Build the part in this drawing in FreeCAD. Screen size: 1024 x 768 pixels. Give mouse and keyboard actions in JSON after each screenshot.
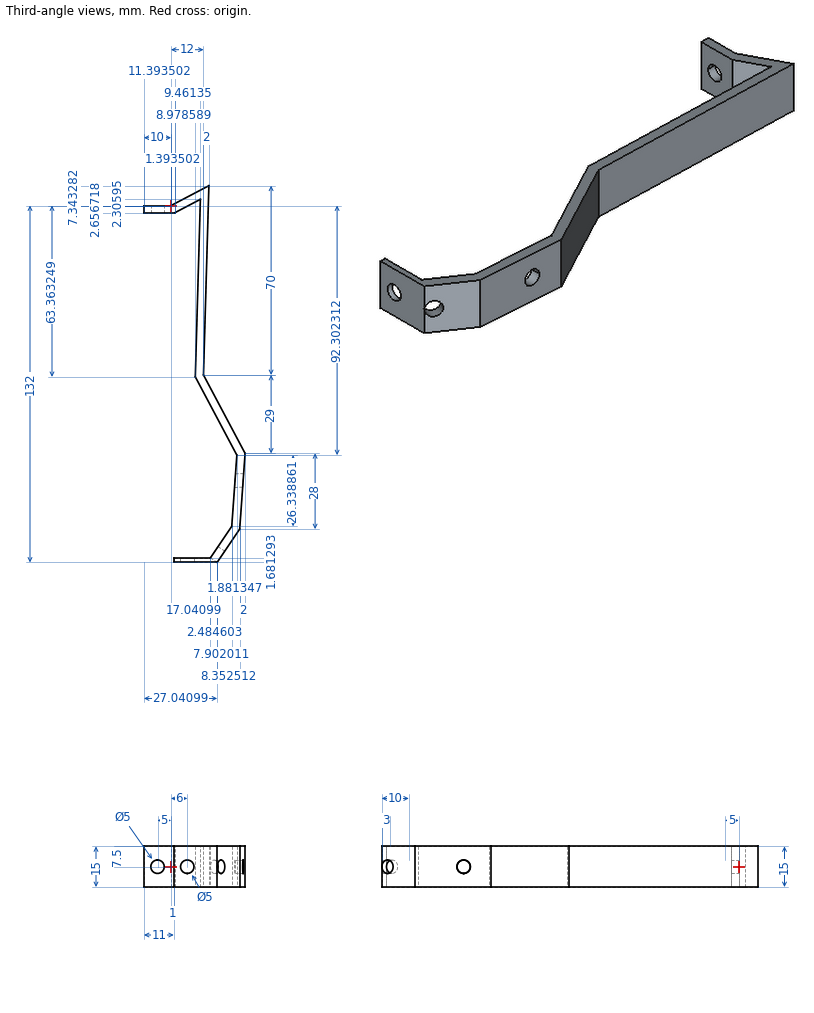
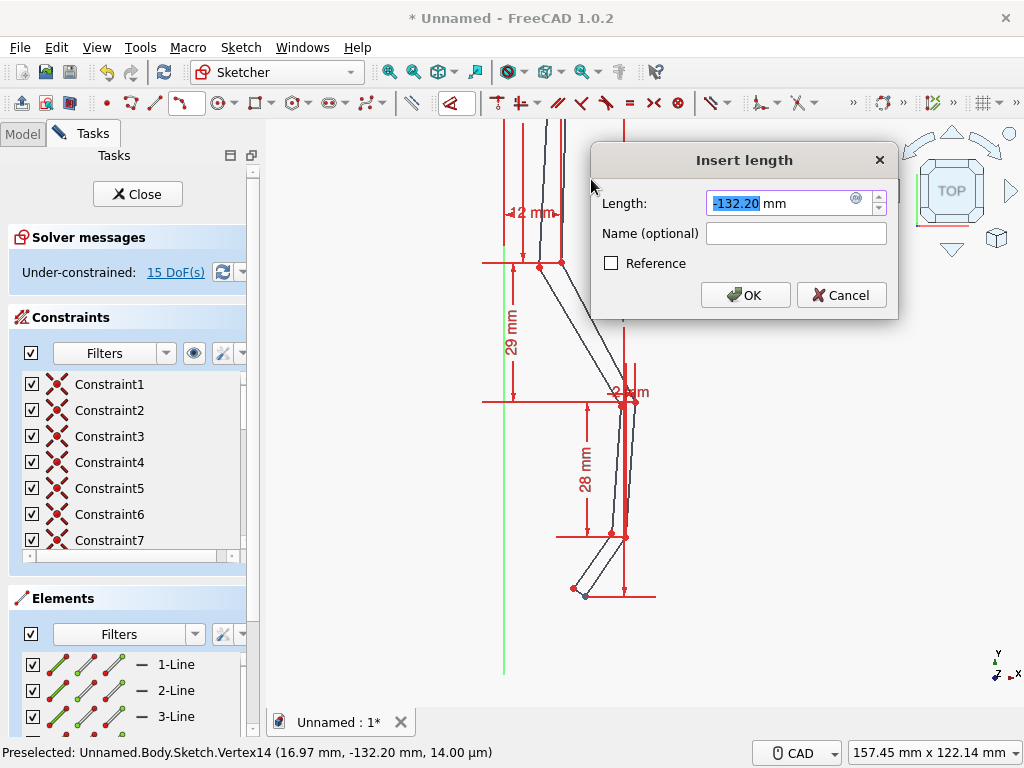
{"action": "type", "text": "-132"}
{"action": "key", "text": "Return"}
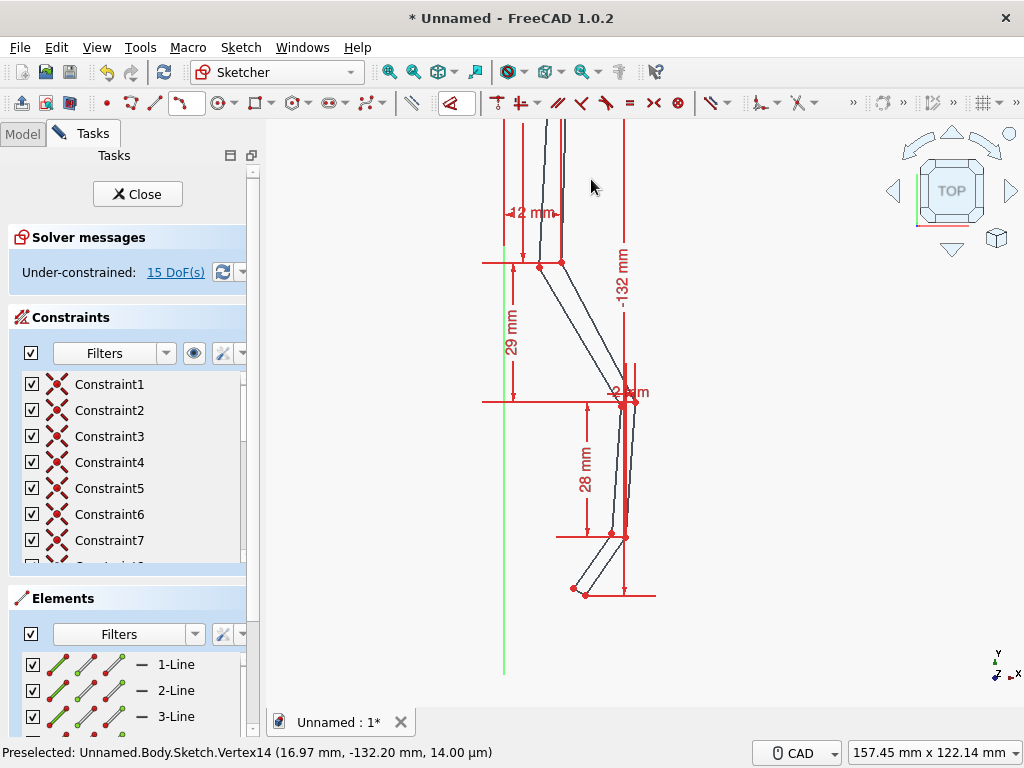
{"action": "scroll", "coordinate": [585, 599], "scroll_direction": "down", "scroll_amount": 3}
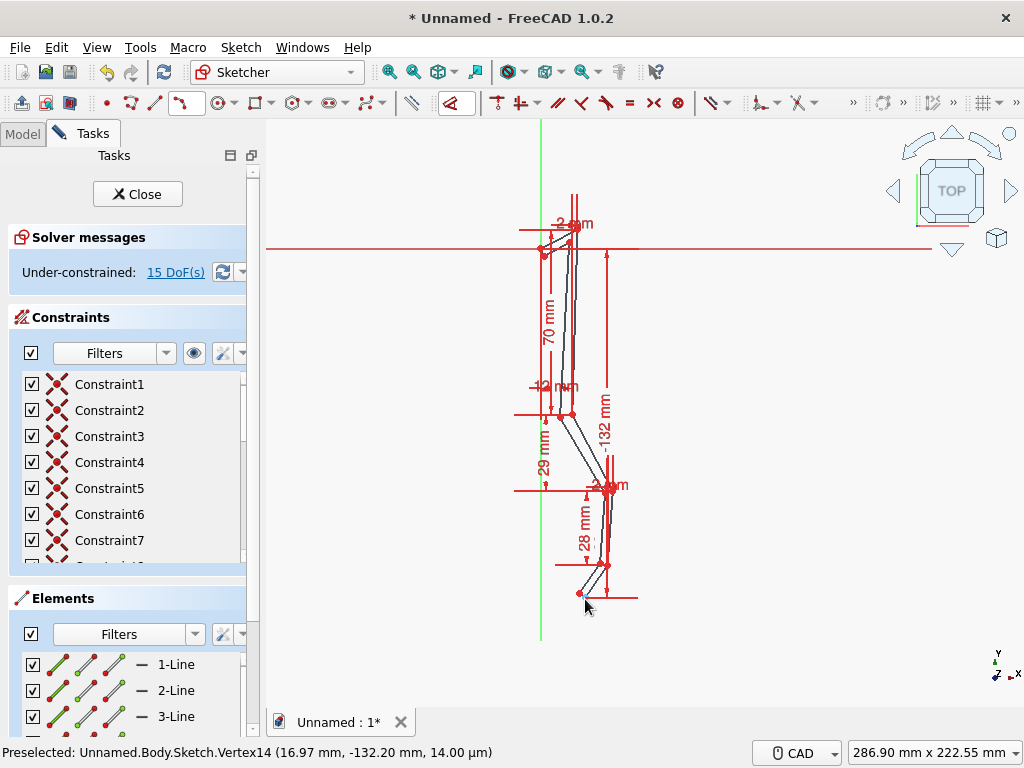
{"action": "scroll", "coordinate": [569, 243], "scroll_direction": "up", "scroll_amount": 10}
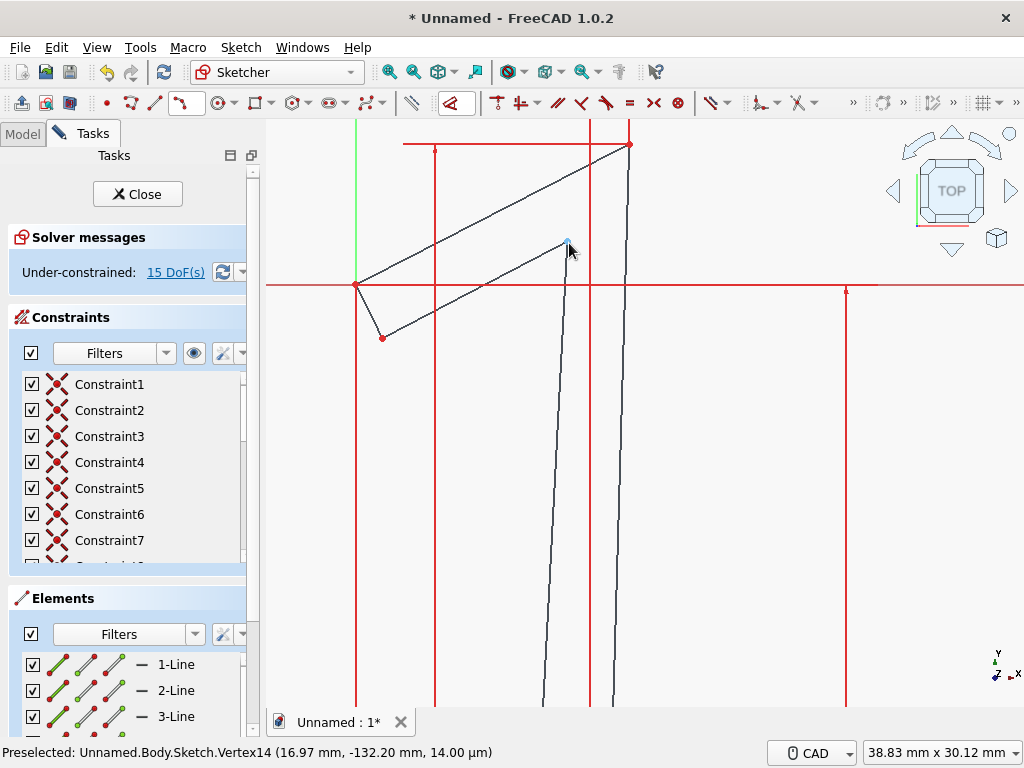
{"action": "left_click", "coordinate": [567, 241]}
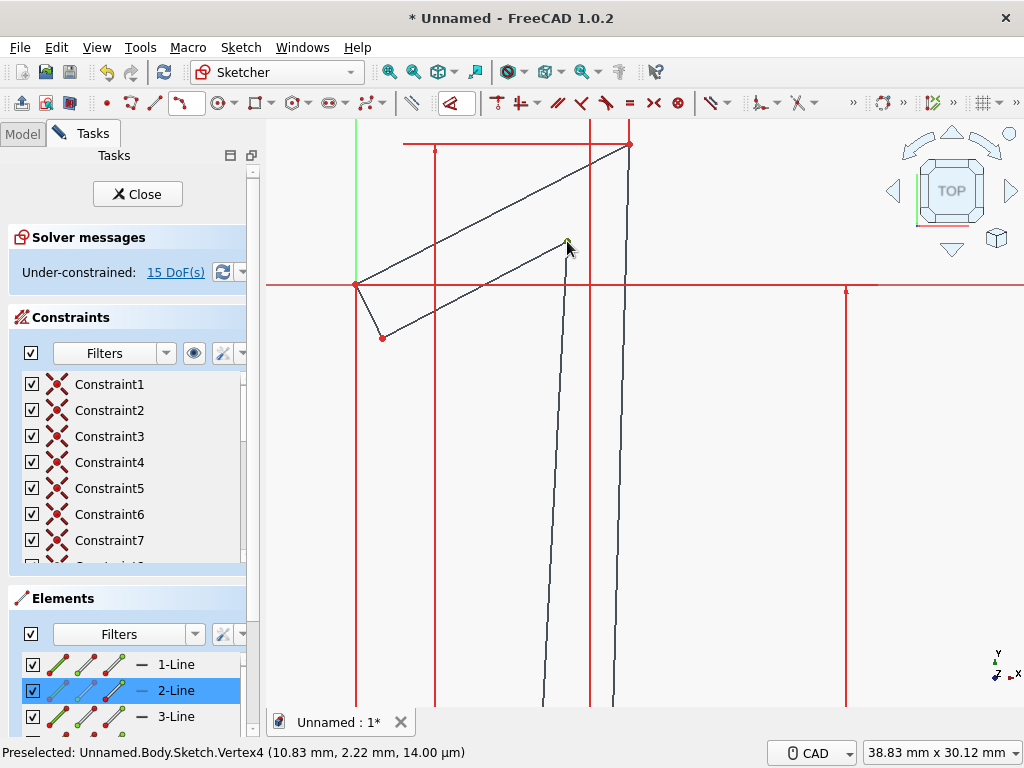
{"action": "key", "text": "i"}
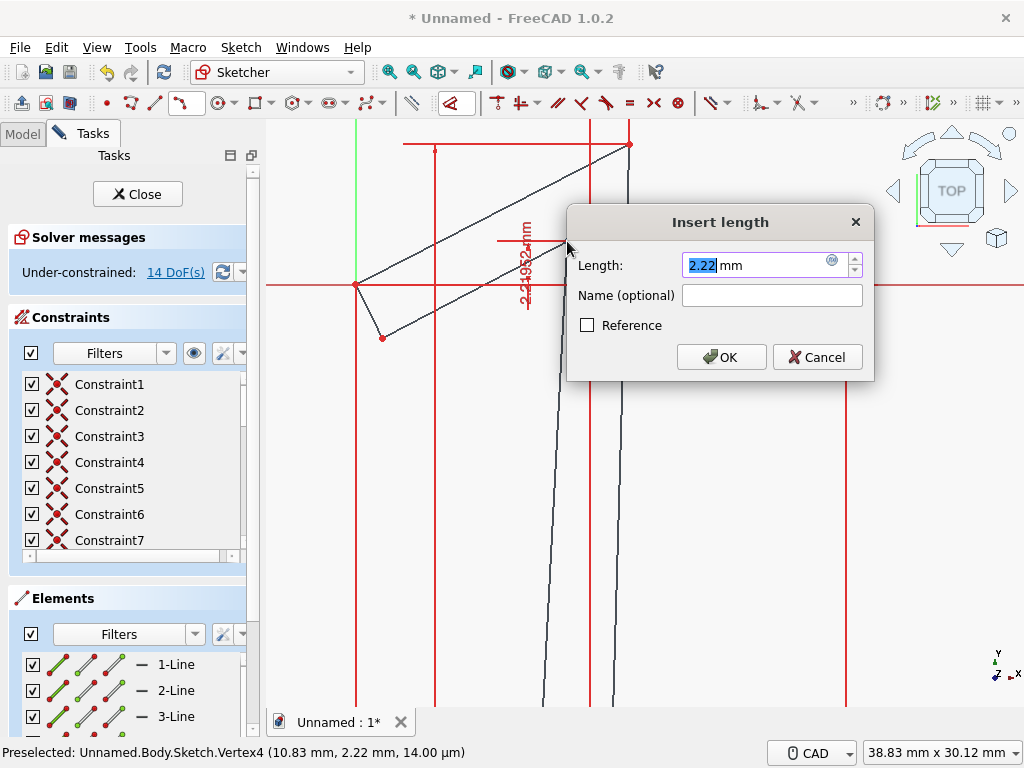
{"action": "type", "text": "2.30595"}
{"action": "key", "text": "Return"}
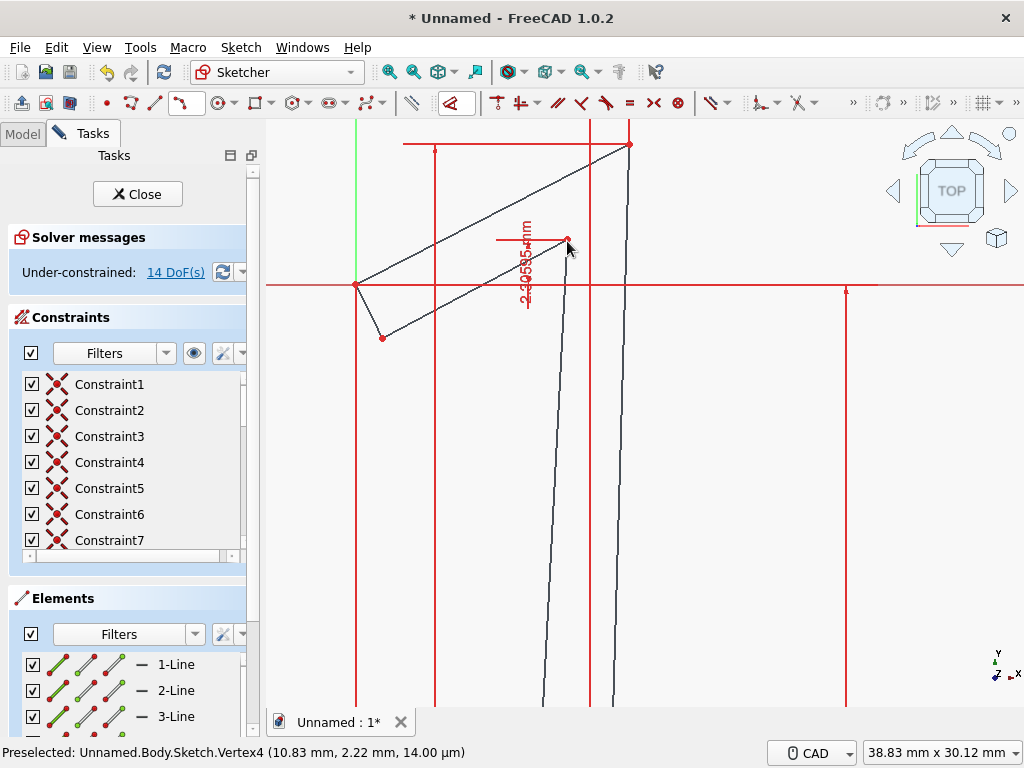
{"action": "left_click", "coordinate": [438, 309]}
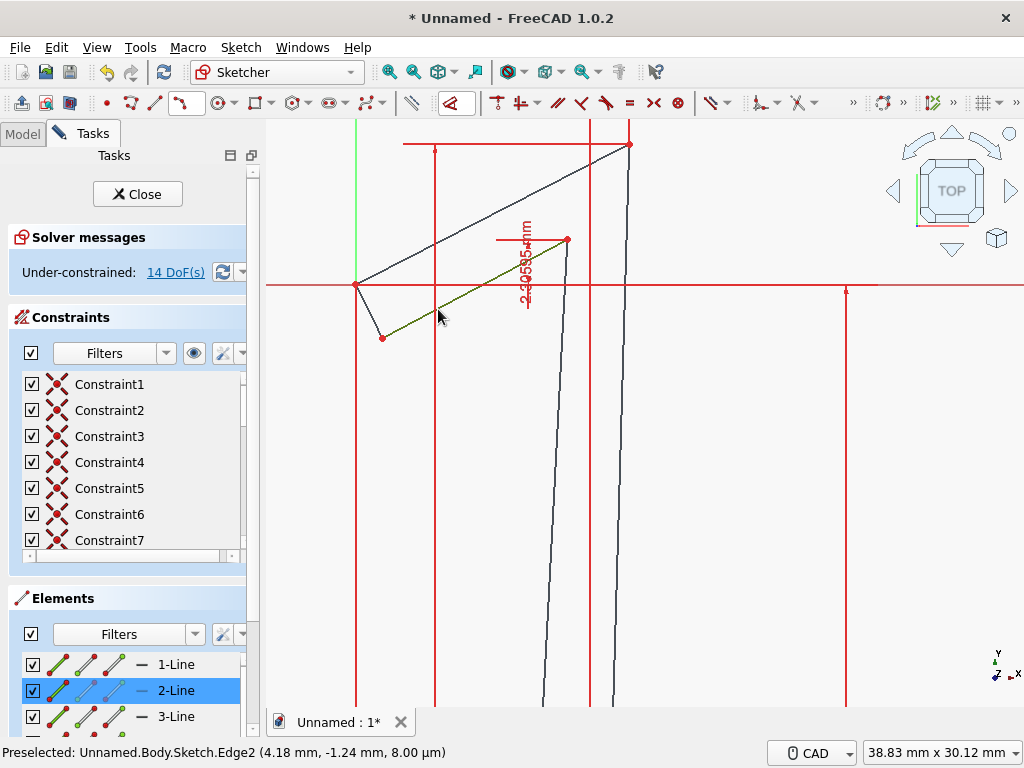
{"action": "key", "text": "l"}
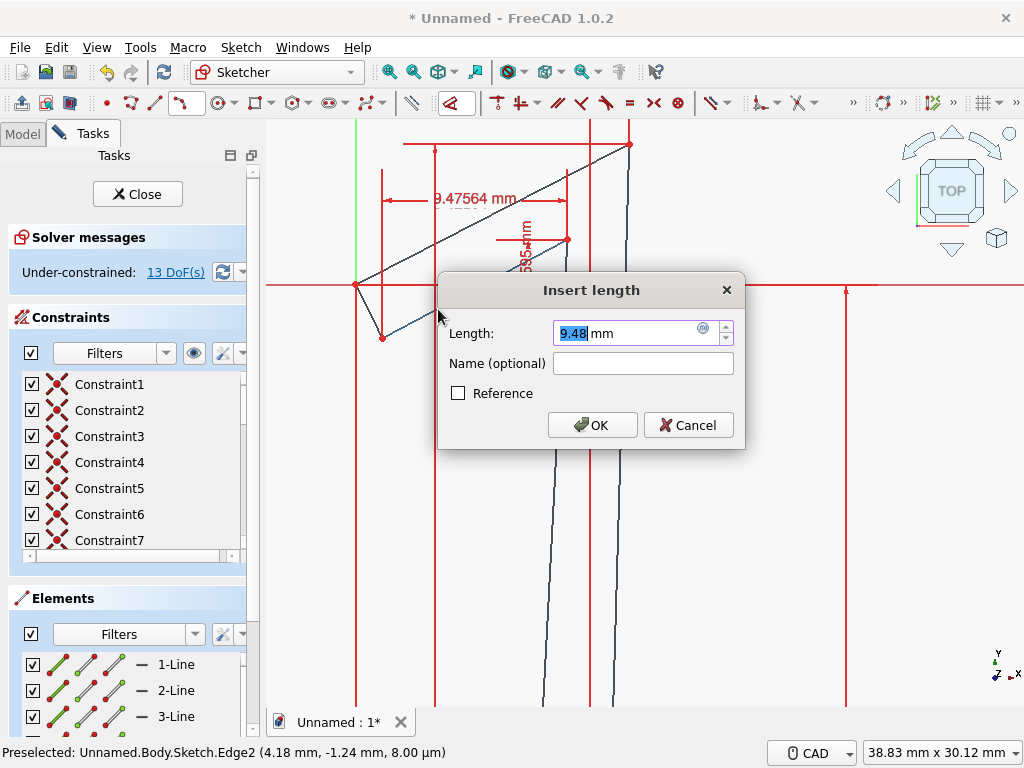
{"action": "type", "text": "9.46135"}
{"action": "key", "text": "Return"}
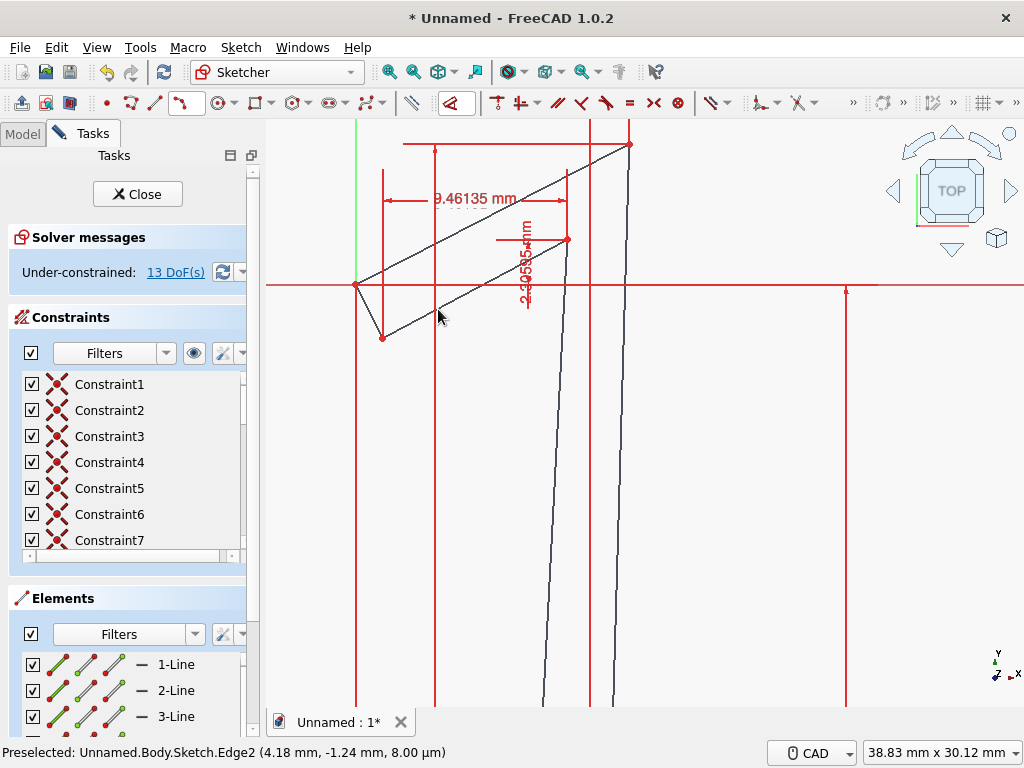
{"action": "scroll", "coordinate": [383, 338], "scroll_direction": "up", "scroll_amount": 2}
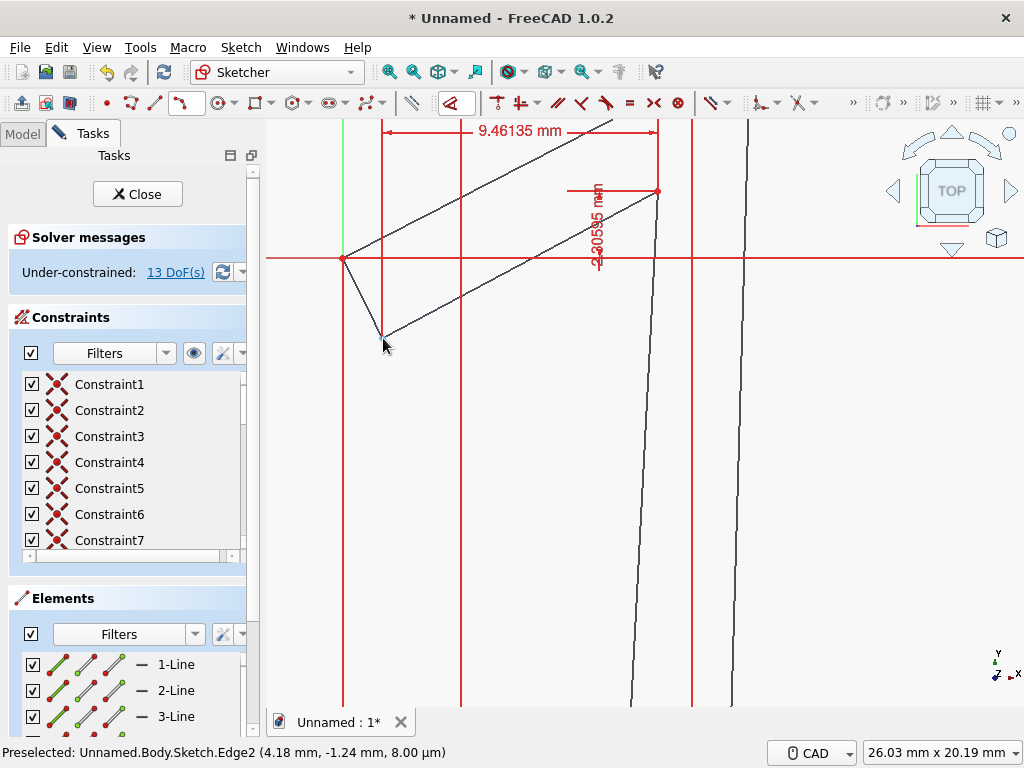
{"action": "left_click", "coordinate": [382, 338]}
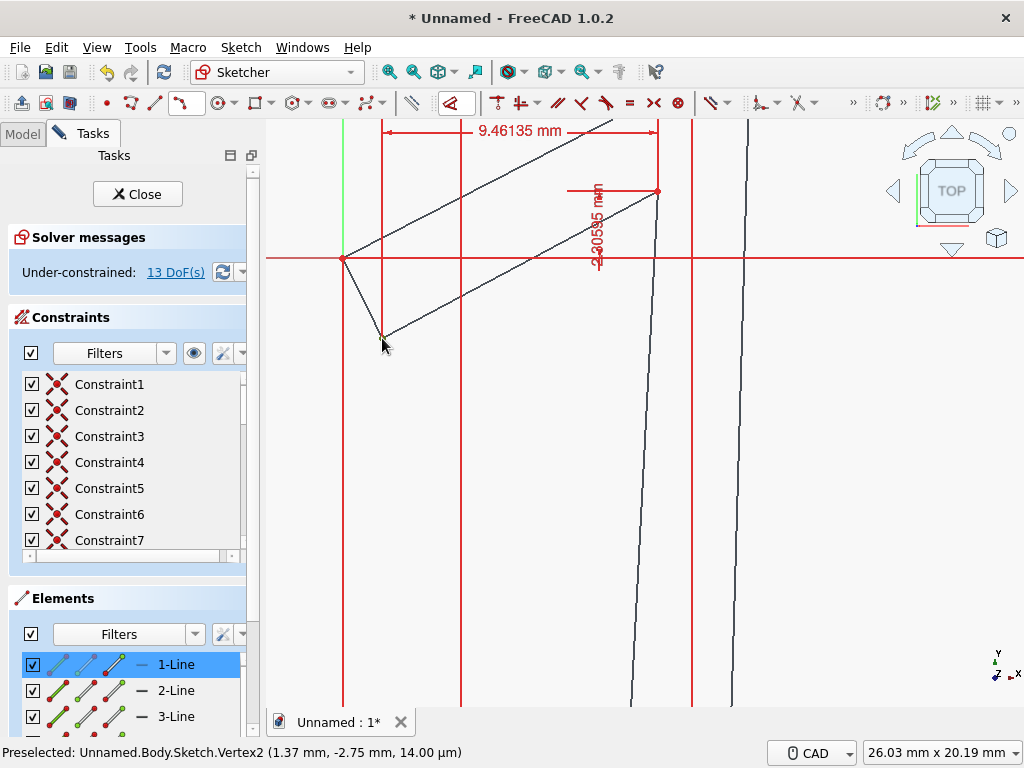
{"action": "left_click", "coordinate": [470, 104]}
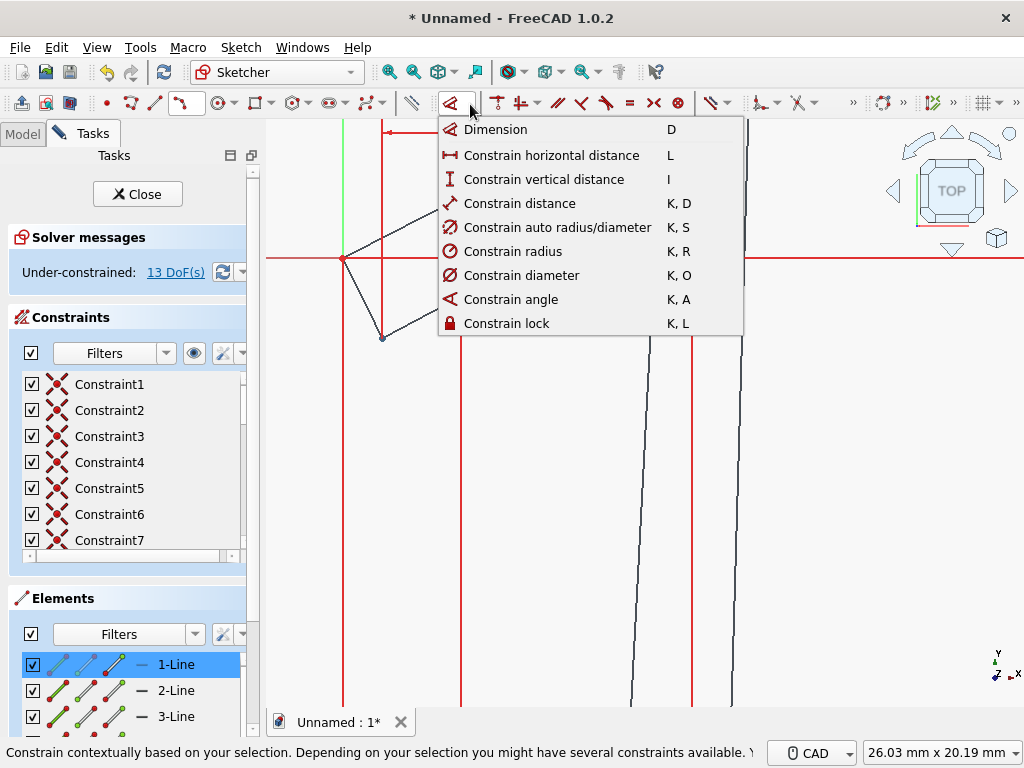
{"action": "left_click", "coordinate": [591, 155]}